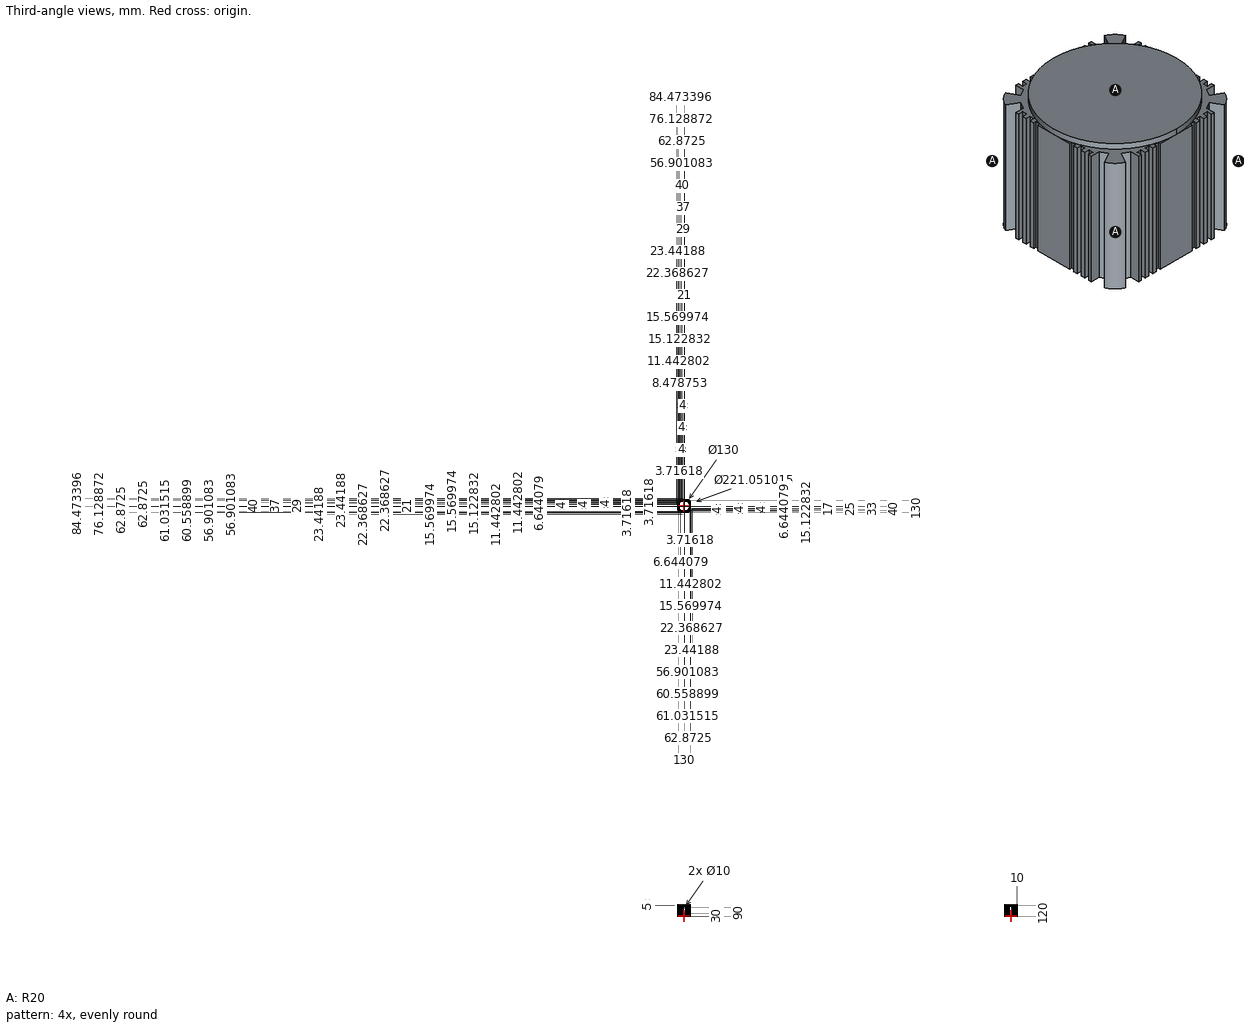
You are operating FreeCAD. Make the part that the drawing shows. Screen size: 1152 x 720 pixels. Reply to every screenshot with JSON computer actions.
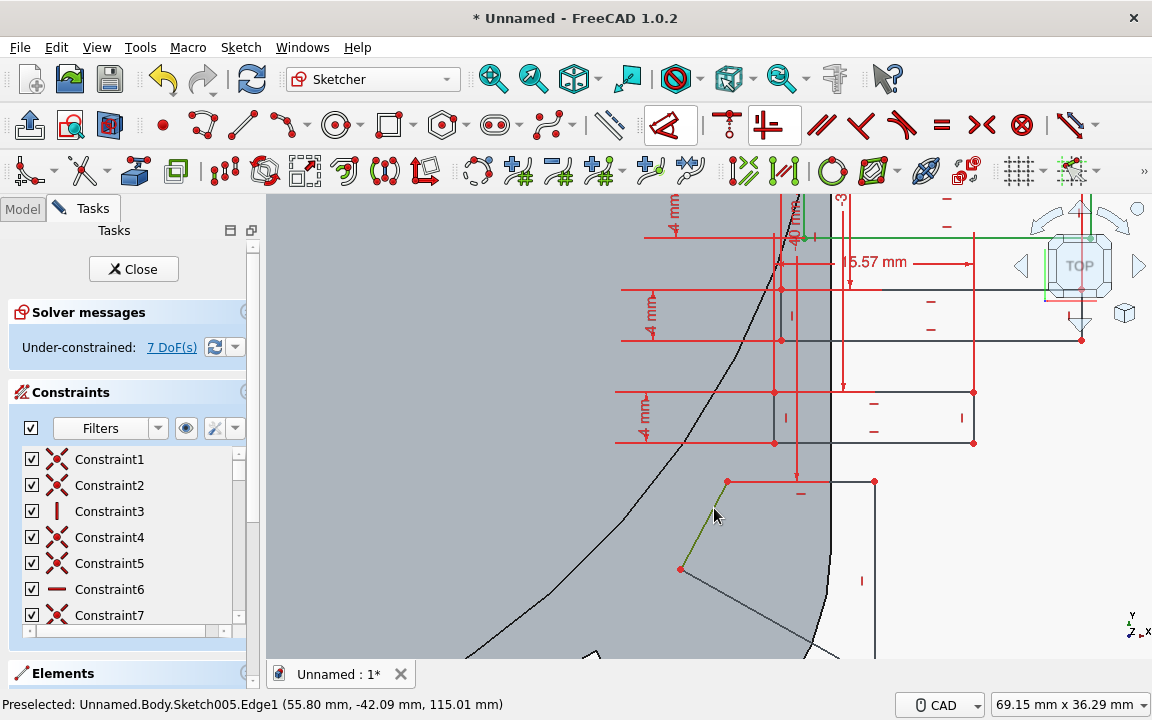
{"action": "left_click", "coordinate": [692, 126]}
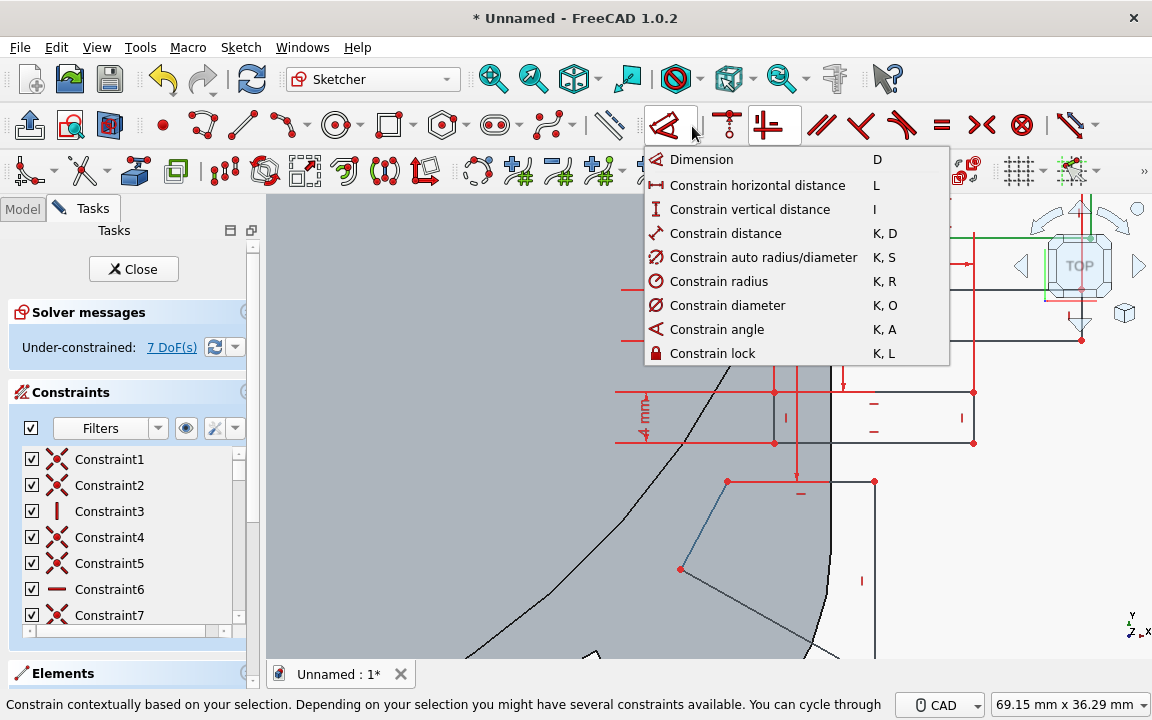
{"action": "left_click", "coordinate": [797, 185]}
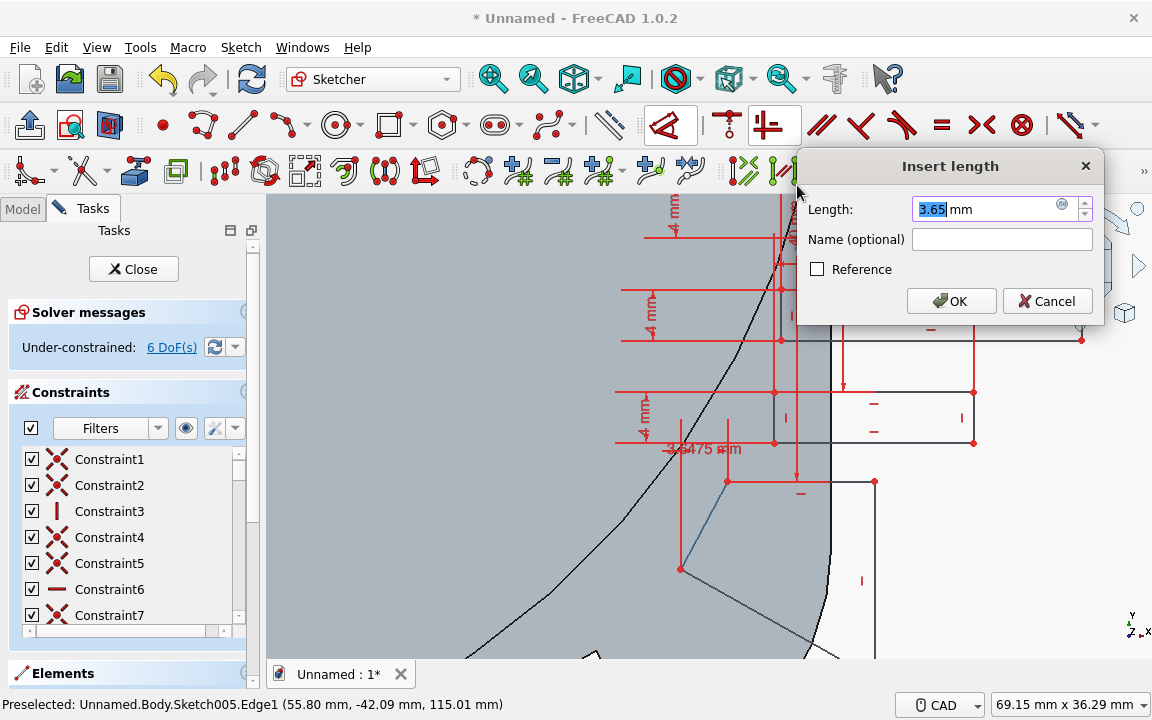
{"action": "type", "text": "3.71618"}
{"action": "key", "text": "Return"}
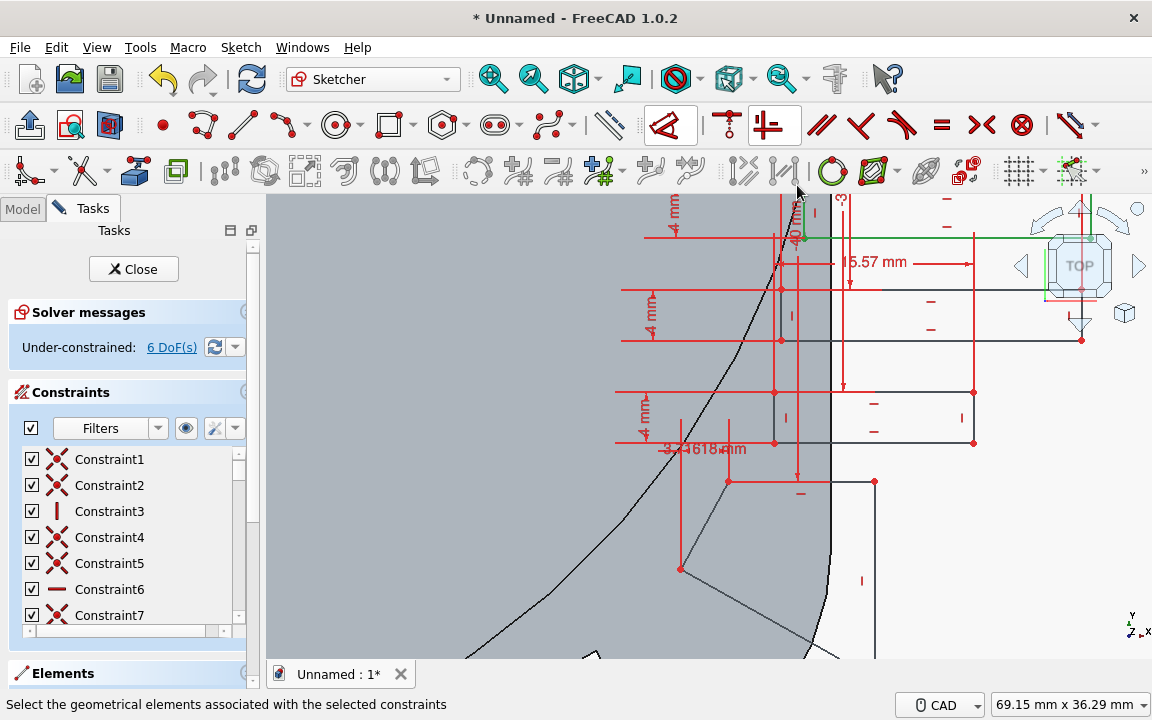
{"action": "left_click", "coordinate": [875, 620]}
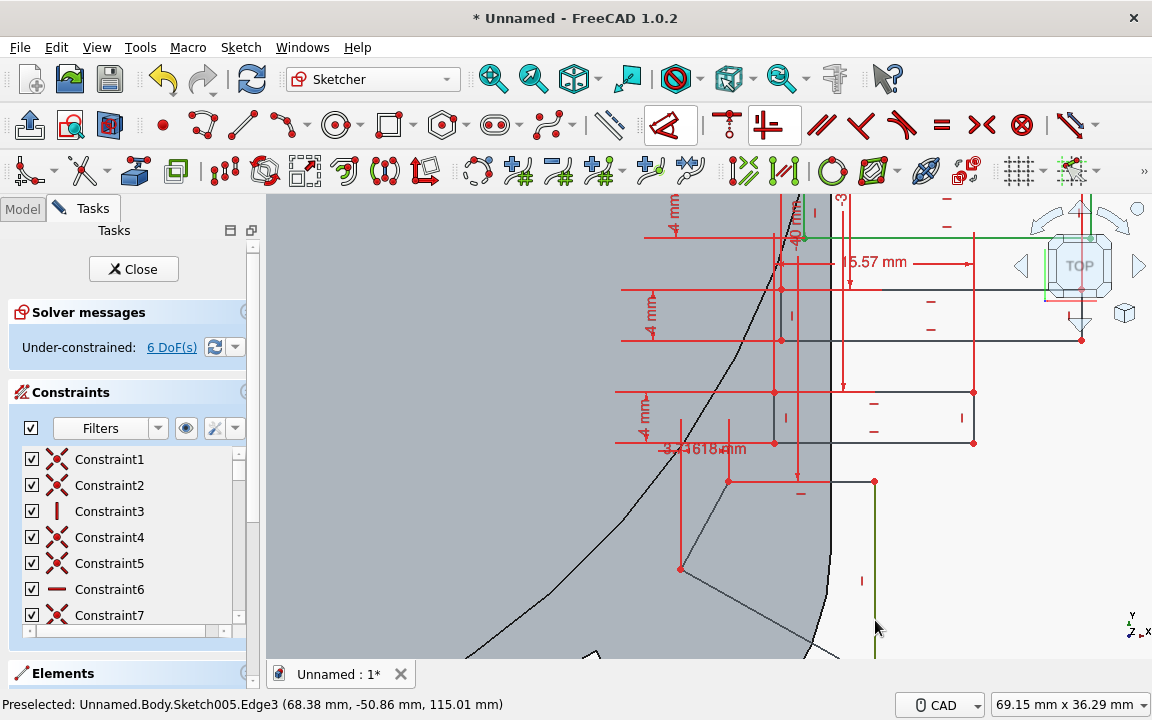
{"action": "key", "text": "i"}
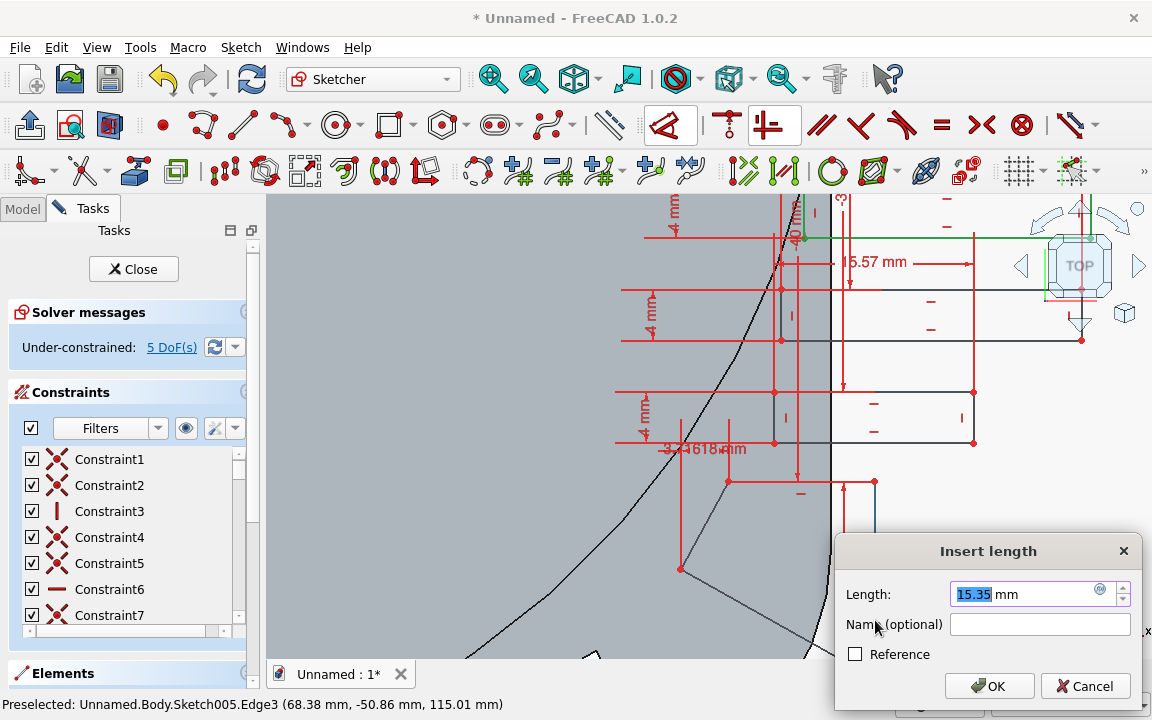
{"action": "type", "text": "15.122832"}
{"action": "key", "text": "Return"}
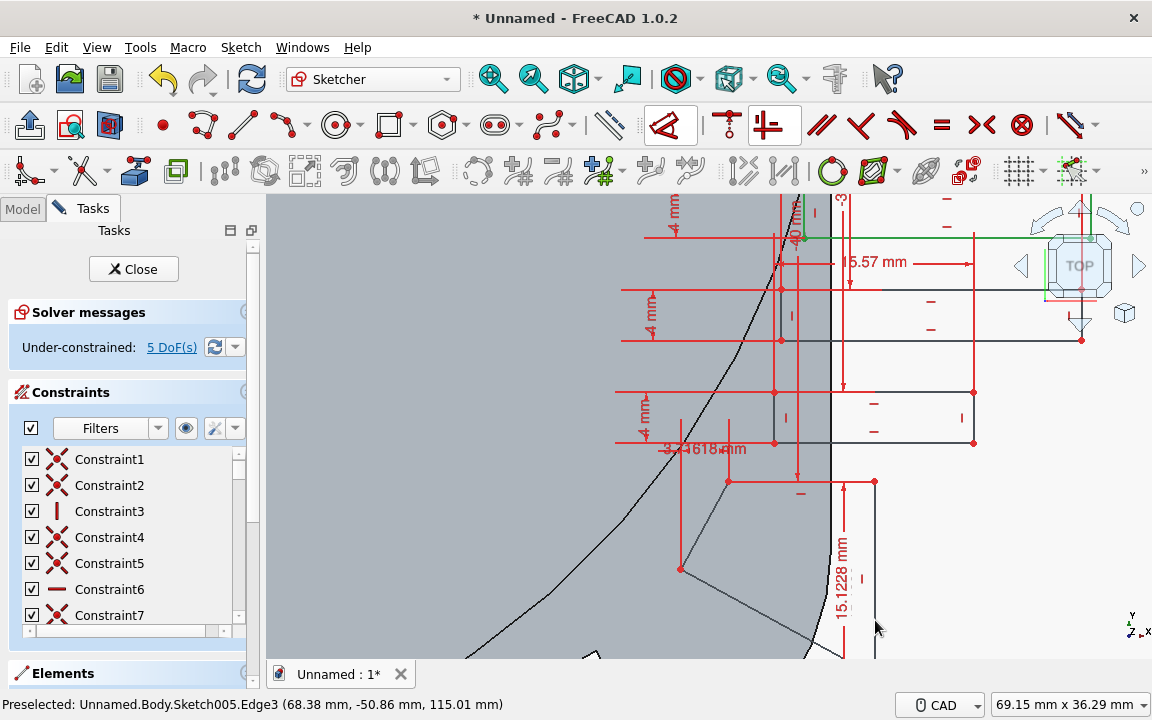
{"action": "left_click", "coordinate": [831, 482]}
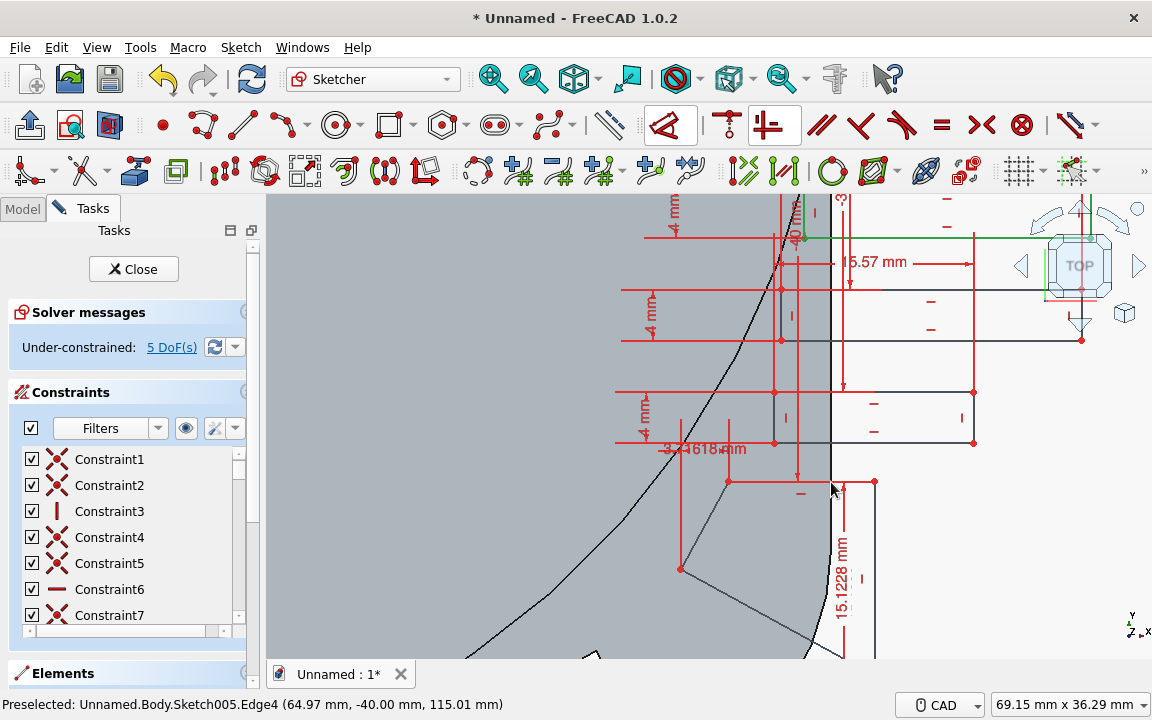
{"action": "left_click", "coordinate": [692, 126]}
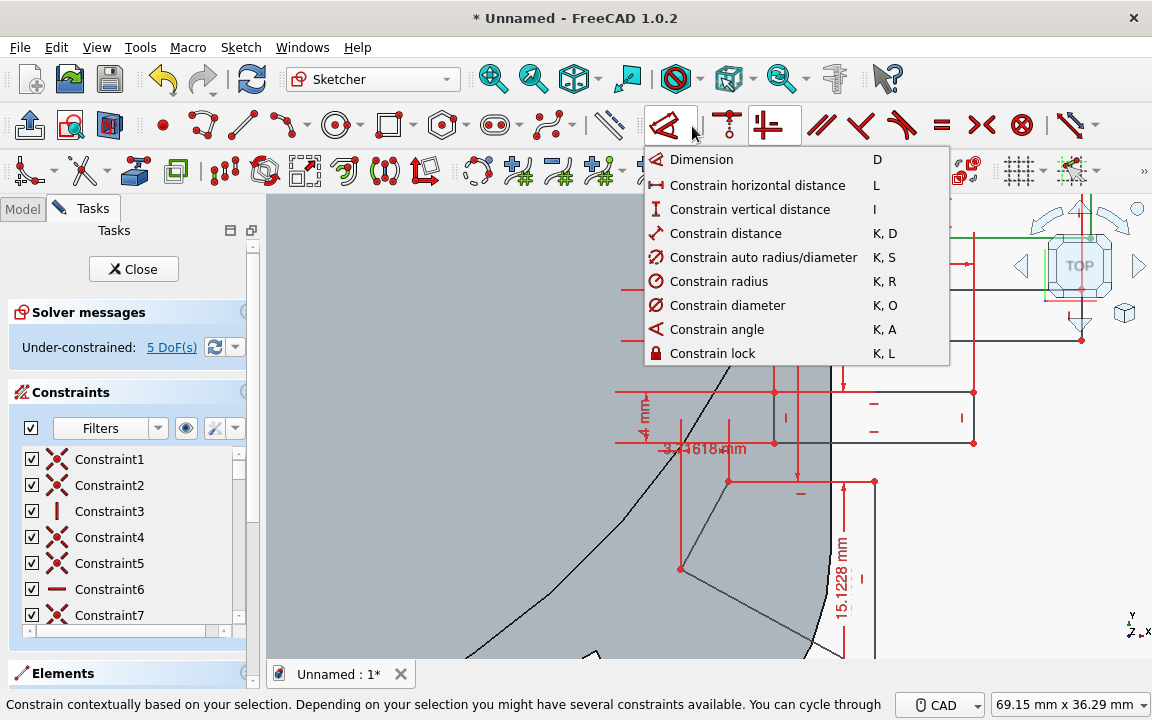
{"action": "left_click", "coordinate": [797, 185]}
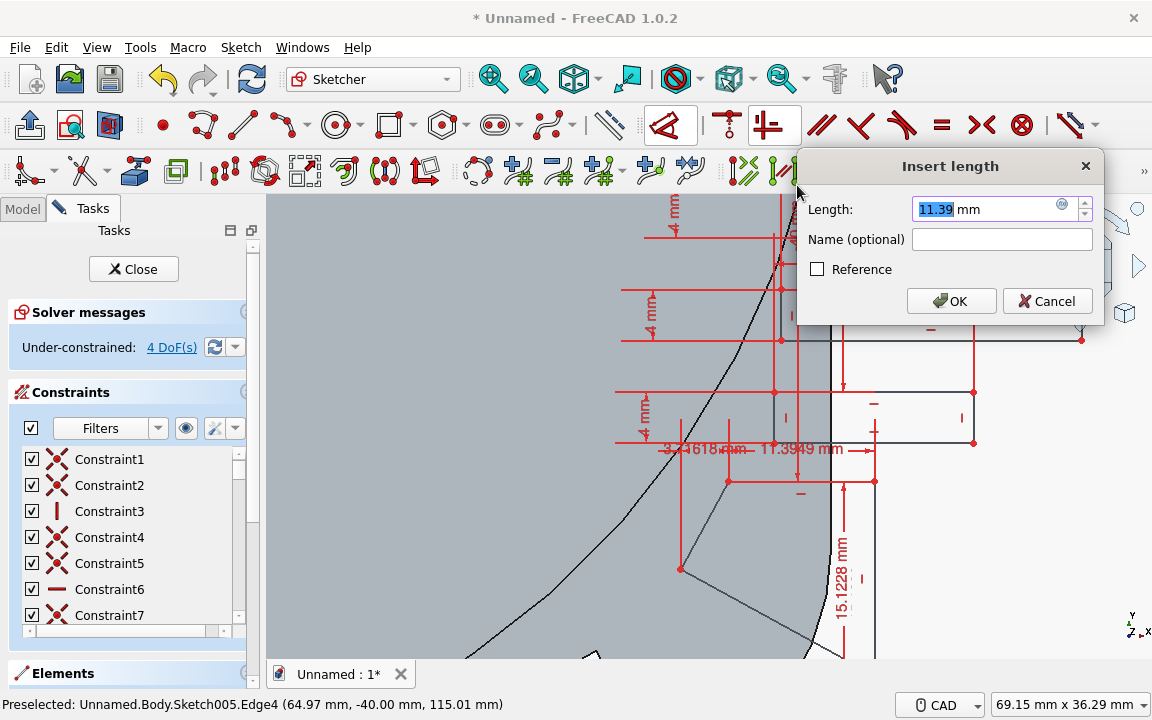
{"action": "type", "text": "11.442802"}
{"action": "key", "text": "Return"}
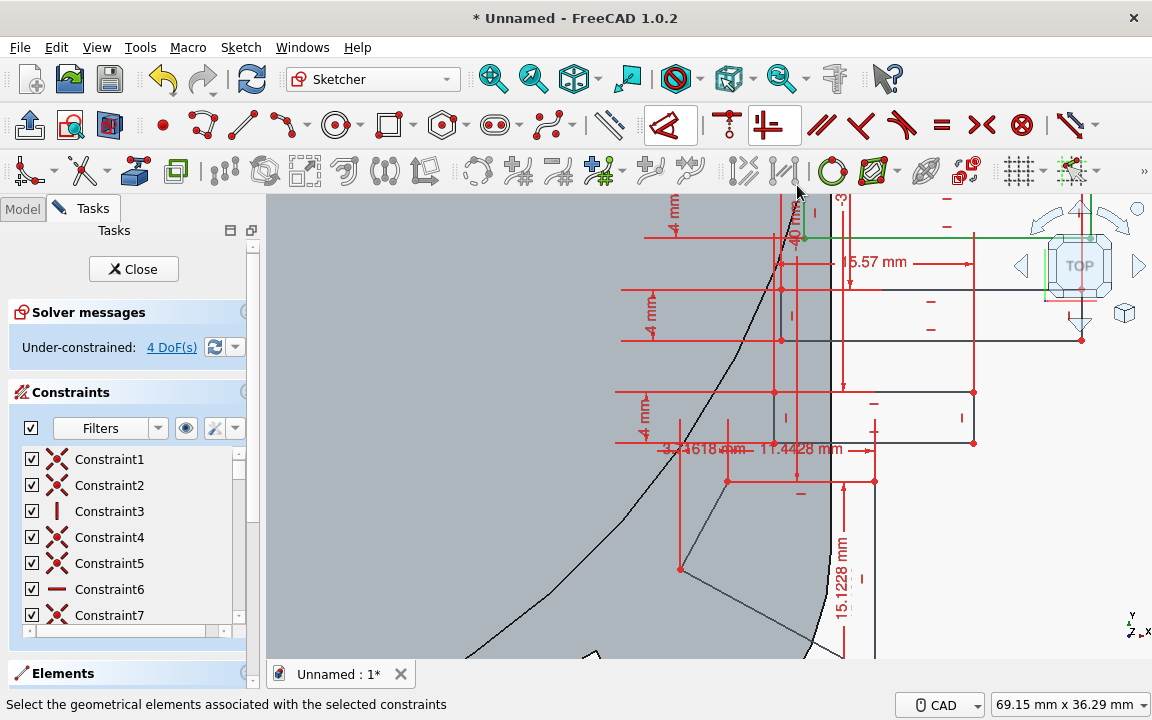
{"action": "left_click", "coordinate": [714, 508]}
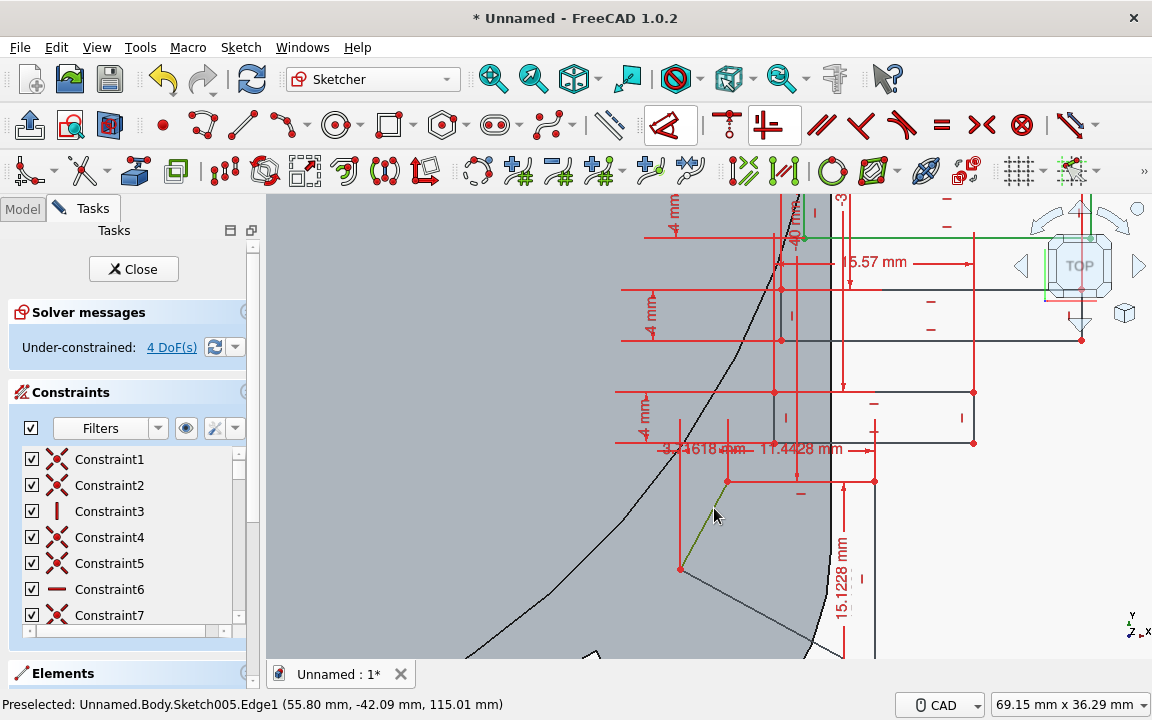
{"action": "left_click", "coordinate": [692, 126]}